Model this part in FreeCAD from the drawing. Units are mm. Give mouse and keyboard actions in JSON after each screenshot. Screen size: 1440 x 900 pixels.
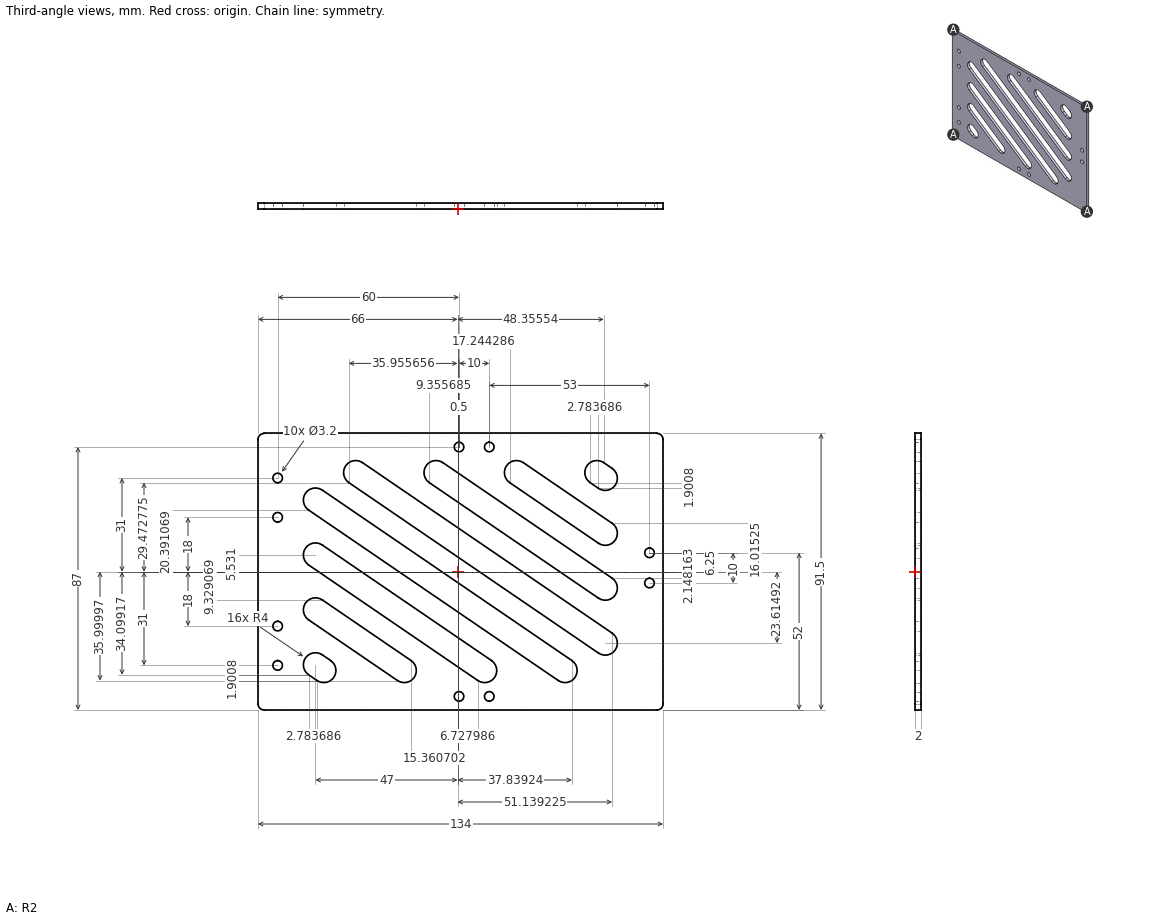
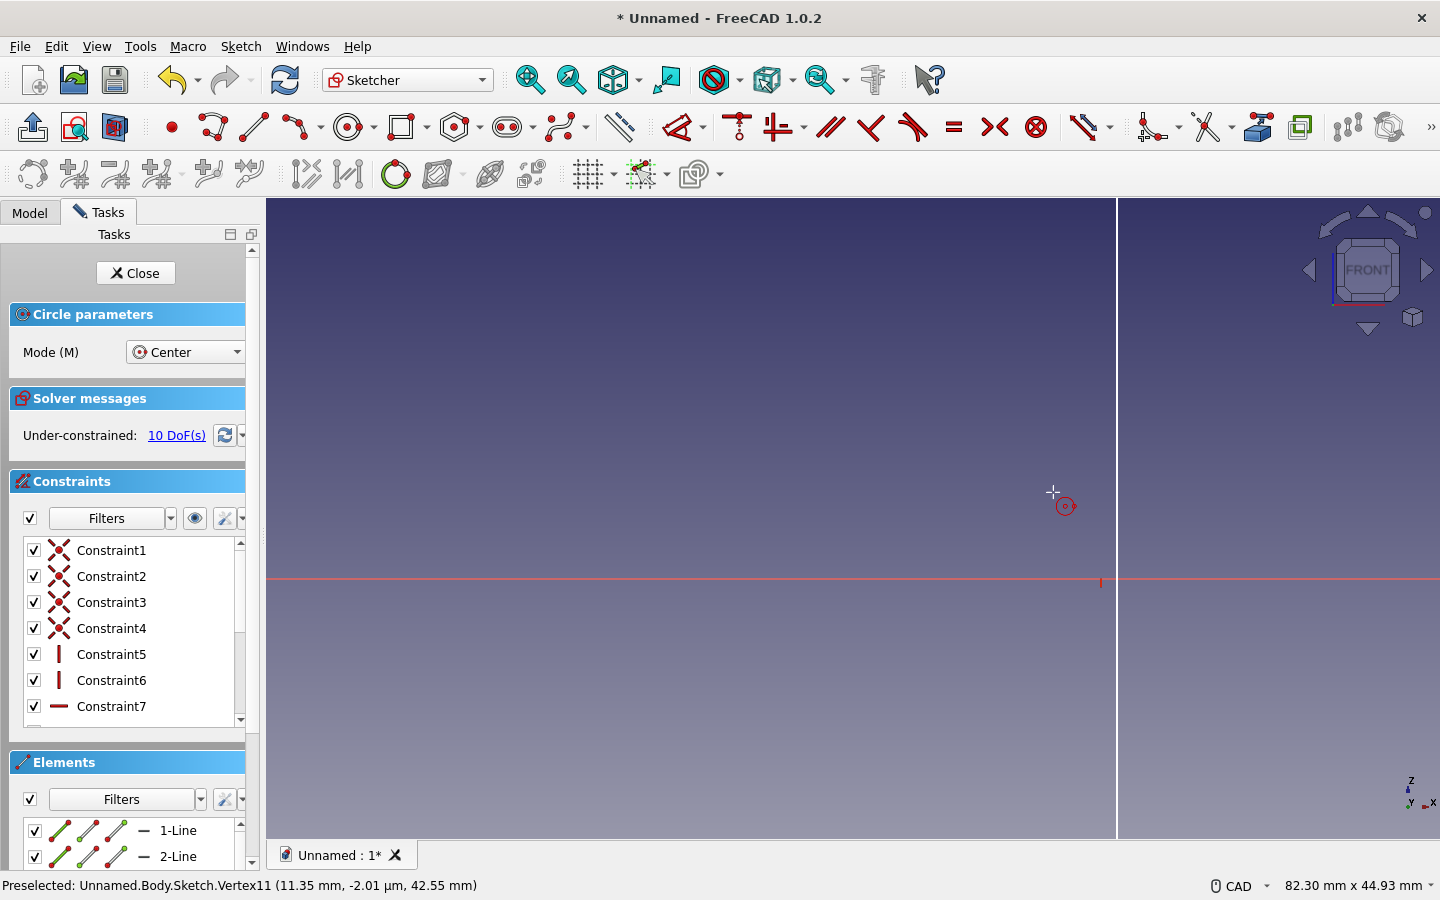
{"action": "left_click", "coordinate": [1052, 490]}
{"action": "mouse_move", "coordinate": [1068, 474]}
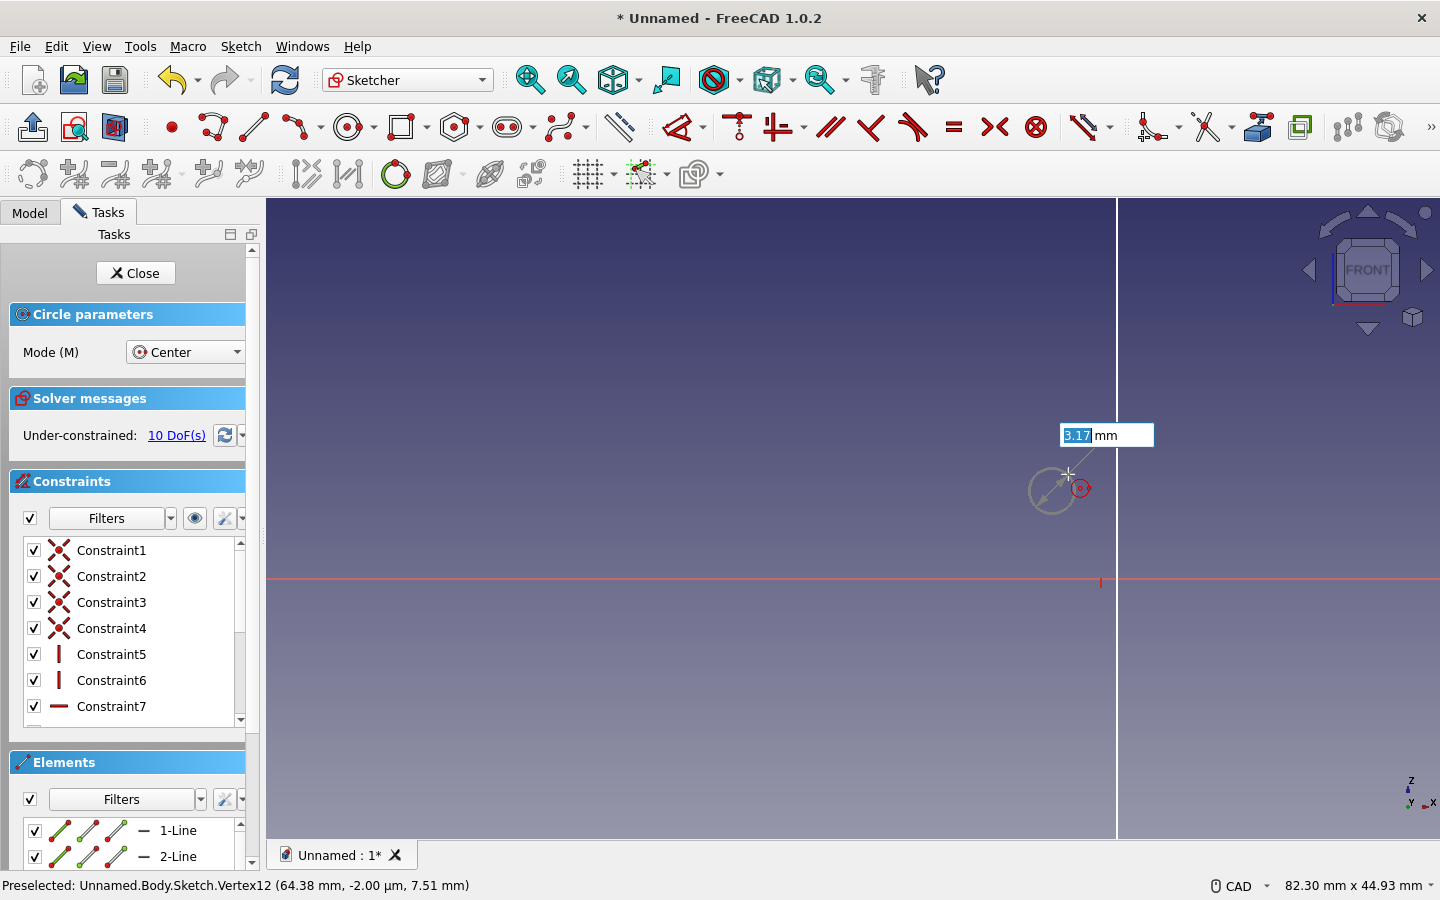
{"action": "type", "text": "3.2"}
{"action": "key", "text": "Return"}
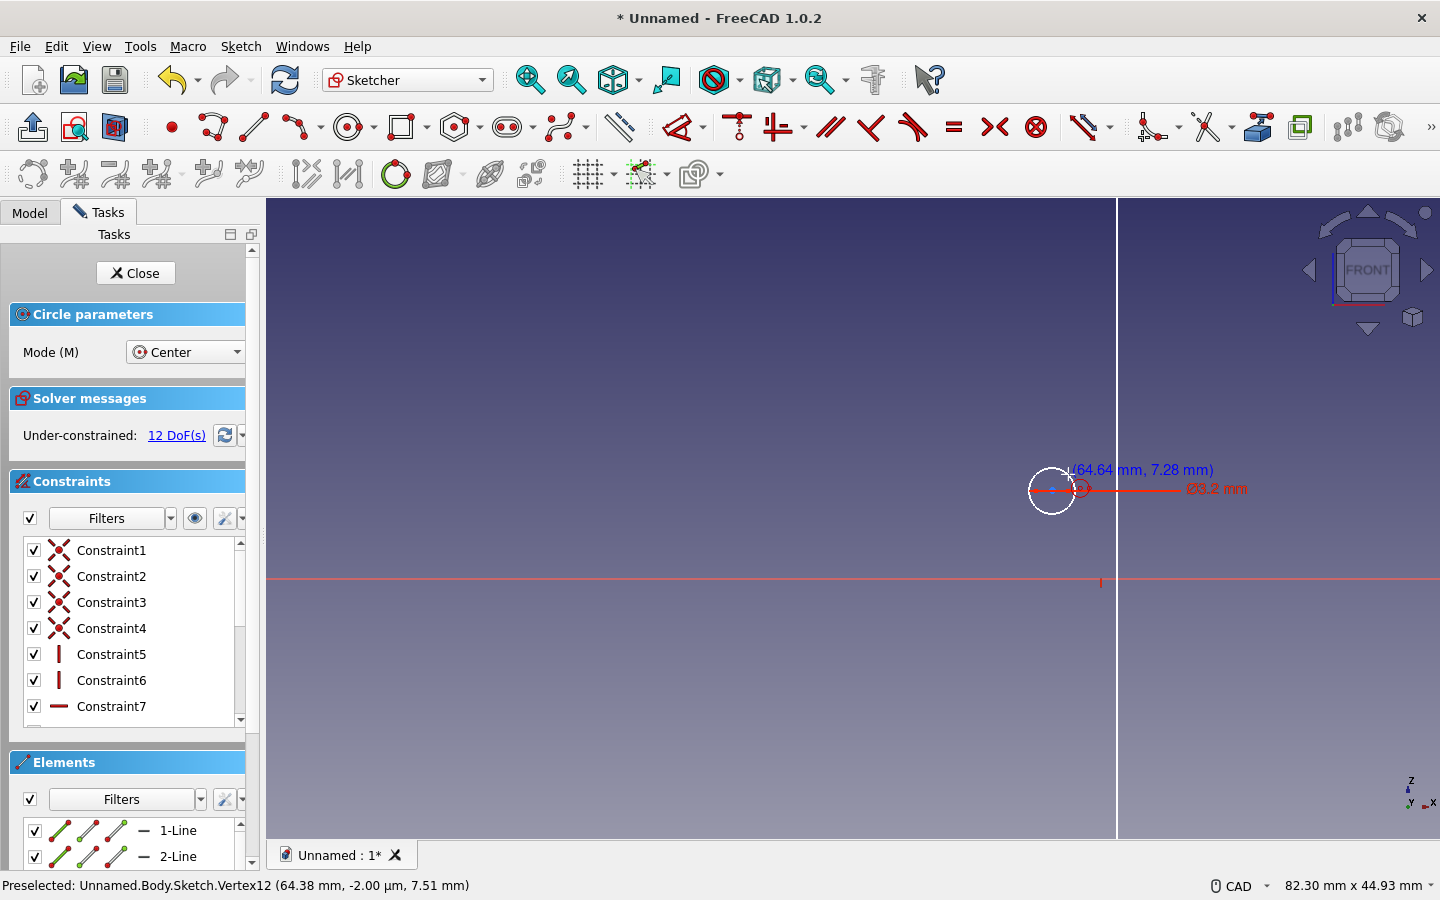
{"action": "scroll", "coordinate": [1054, 492], "scroll_direction": "down", "scroll_amount": 6}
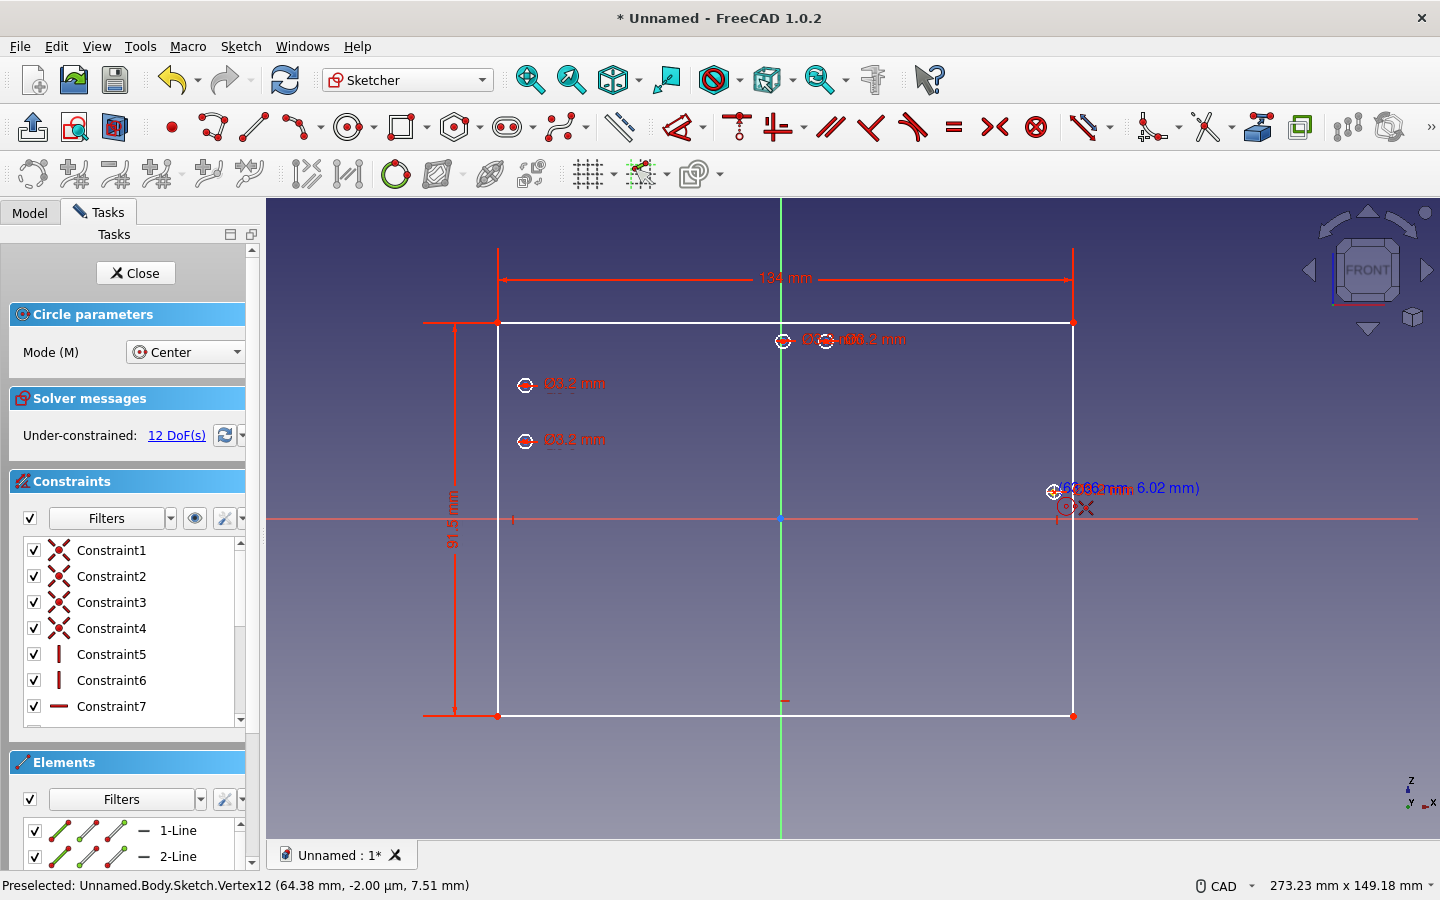
{"action": "scroll", "coordinate": [525, 596], "scroll_direction": "up", "scroll_amount": 6}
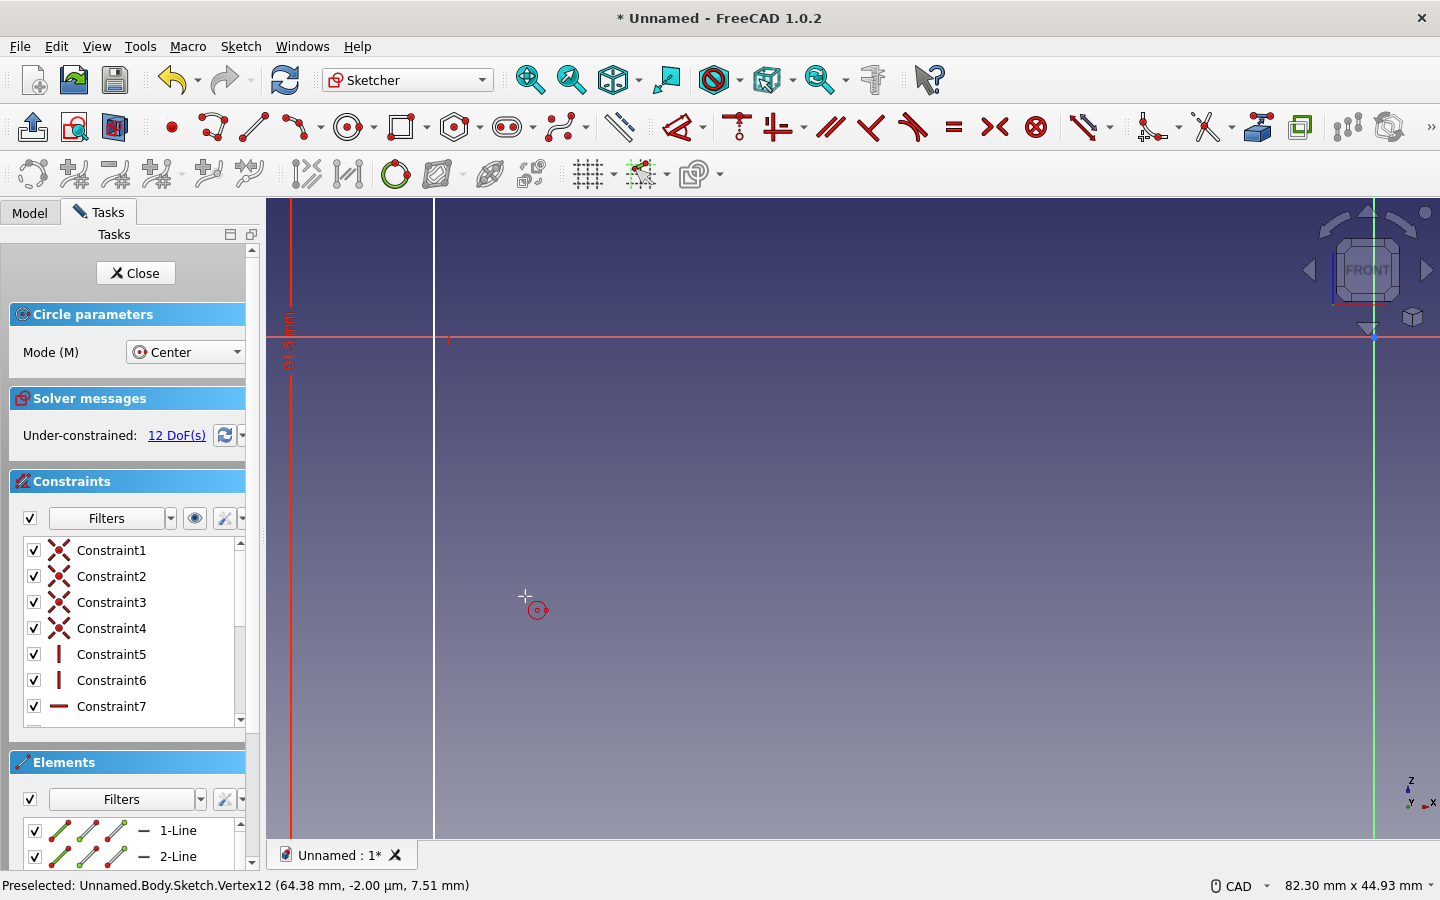
{"action": "left_click", "coordinate": [525, 594]}
{"action": "mouse_move", "coordinate": [542, 578]}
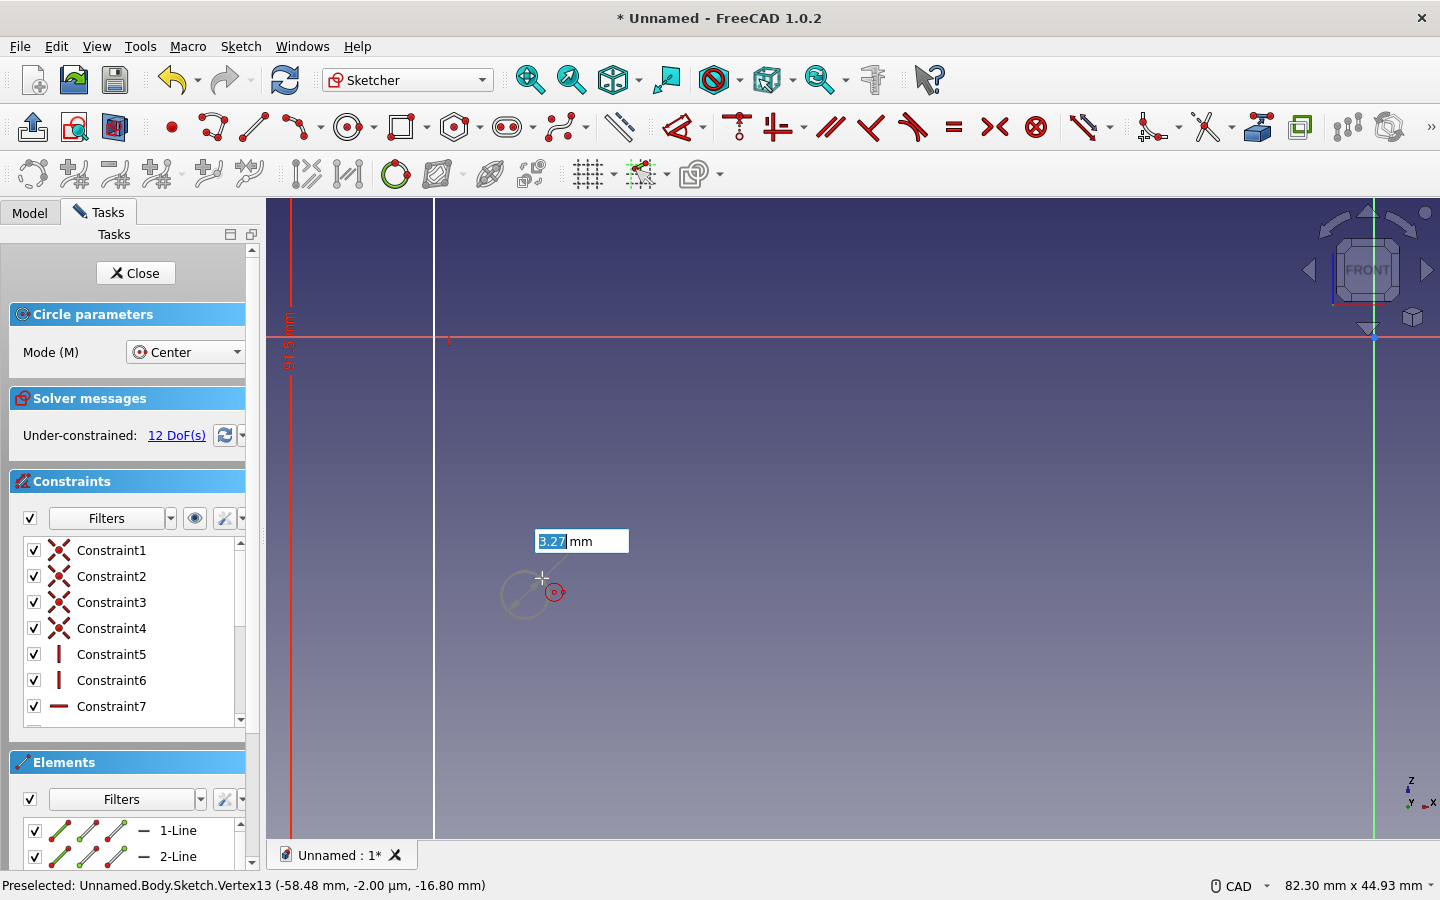
{"action": "type", "text": "3.2"}
{"action": "key", "text": "Return"}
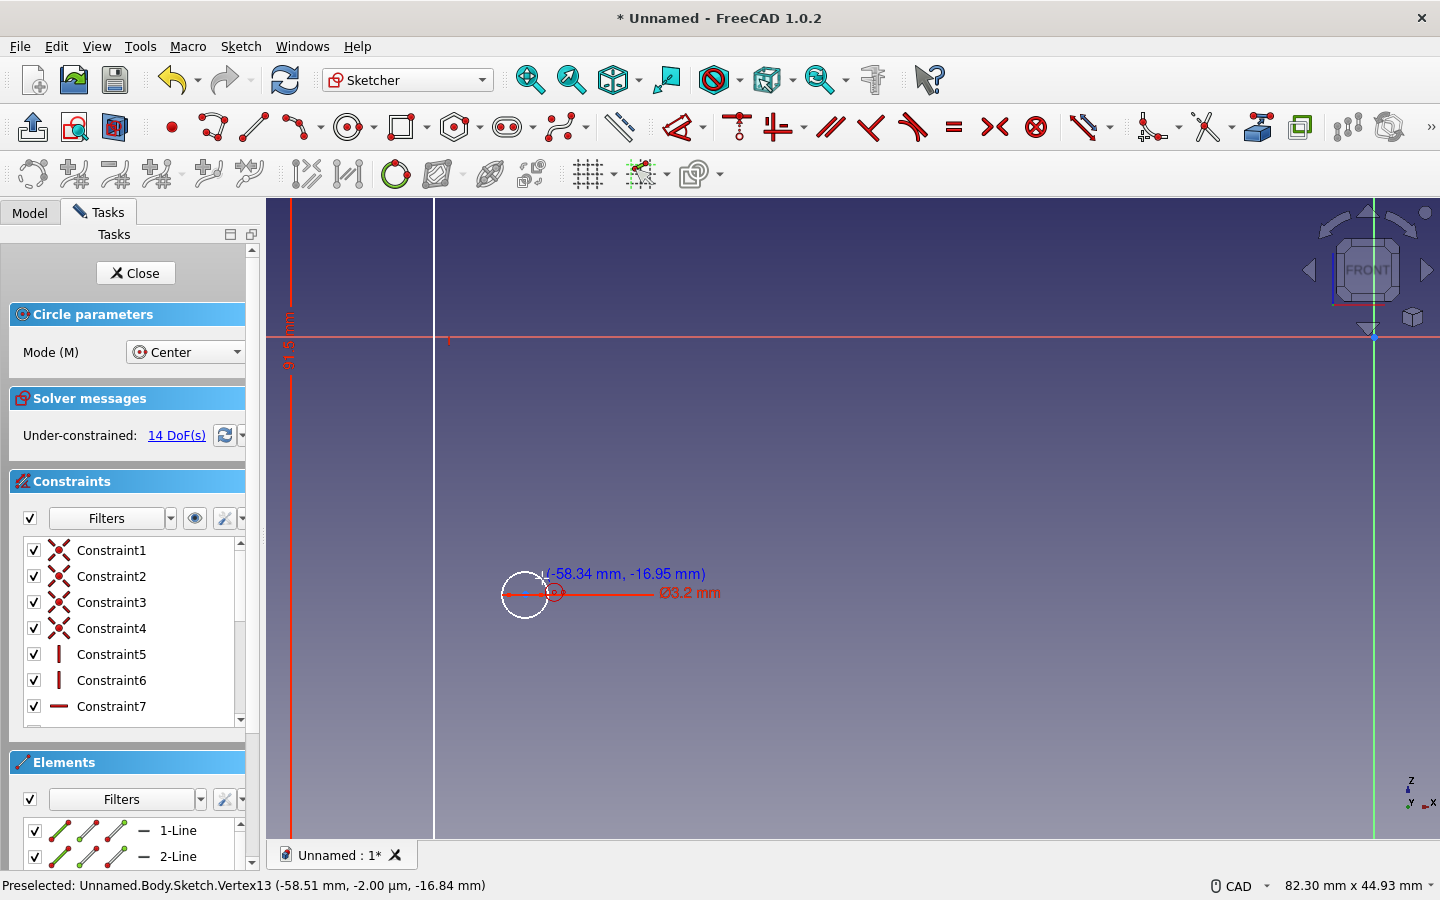
{"action": "left_click", "coordinate": [525, 779]}
{"action": "mouse_move", "coordinate": [542, 763]}